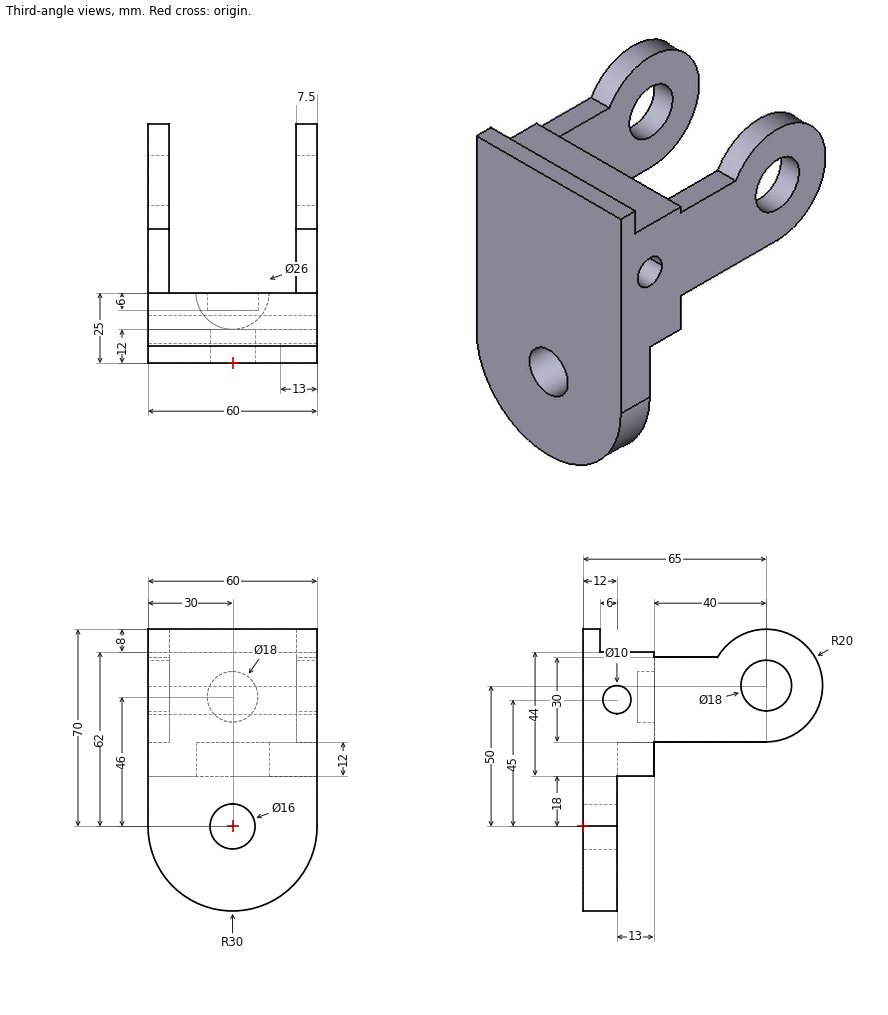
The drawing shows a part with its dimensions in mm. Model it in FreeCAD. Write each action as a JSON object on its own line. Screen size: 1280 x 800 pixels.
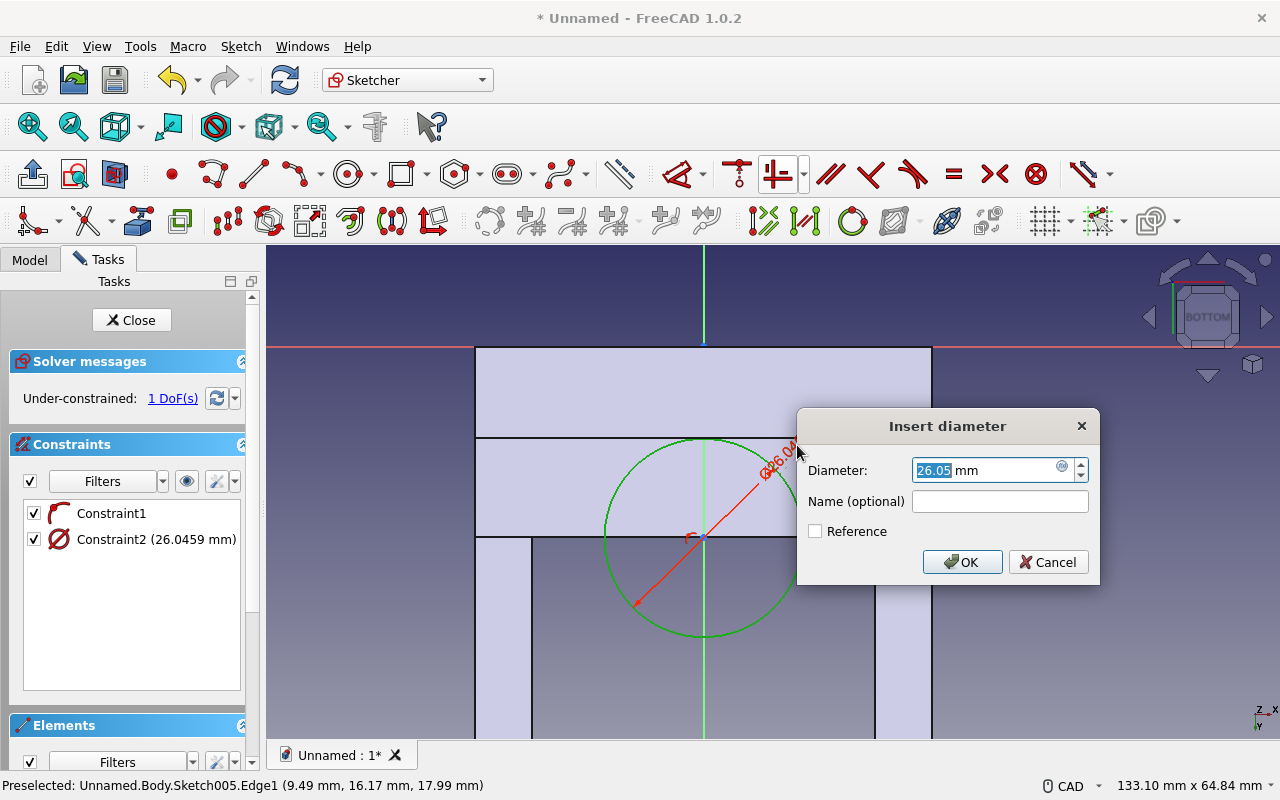
{"action": "type", "text": "26"}
{"action": "key", "text": "Return"}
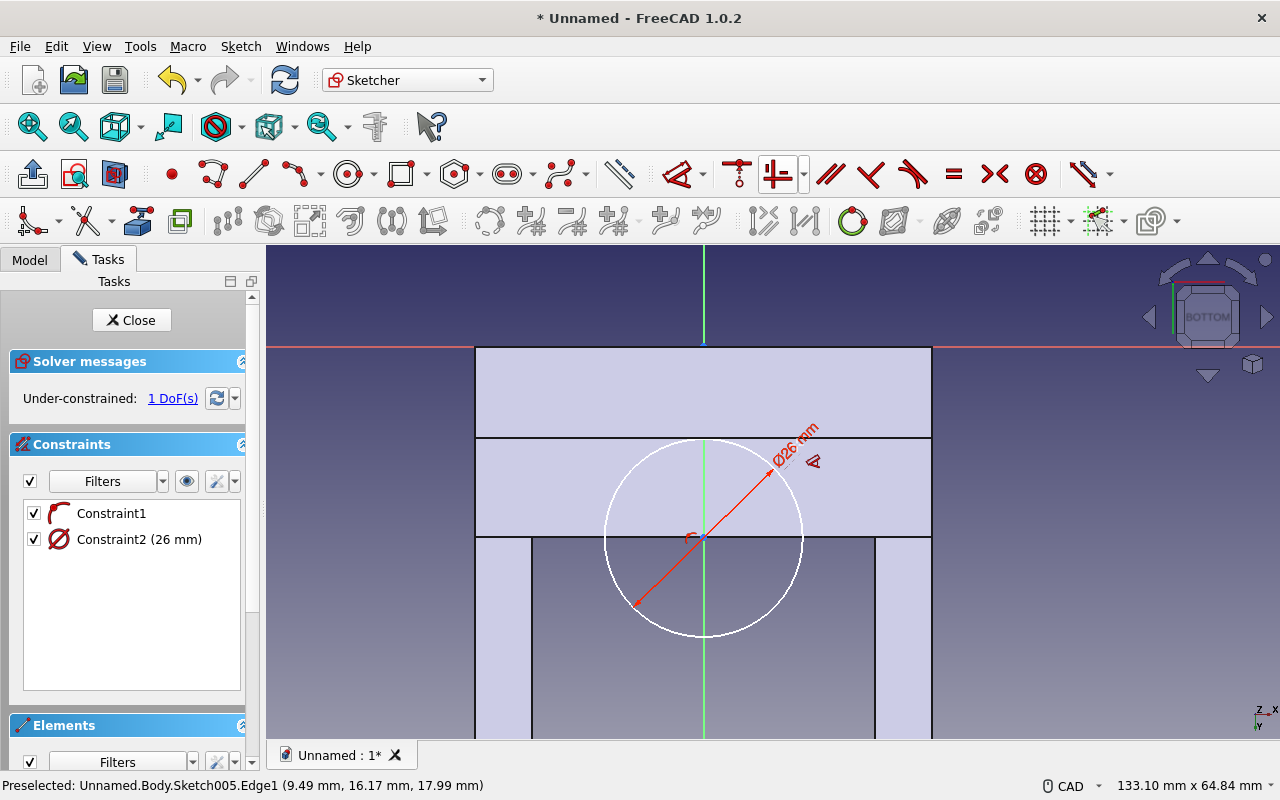
{"action": "left_click", "coordinate": [704, 538]}
{"action": "left_click", "coordinate": [738, 398]}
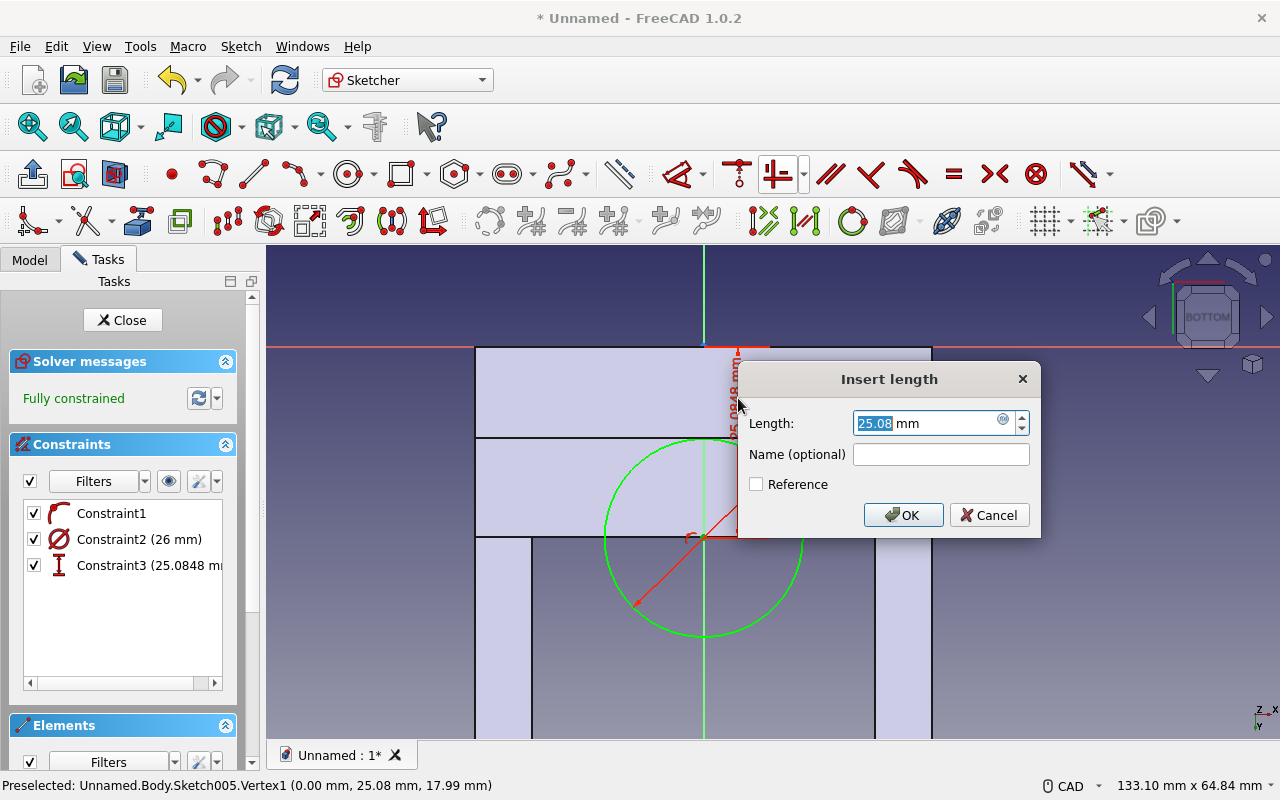
{"action": "type", "text": "25"}
{"action": "key", "text": "Return"}
{"action": "key", "text": "Escape"}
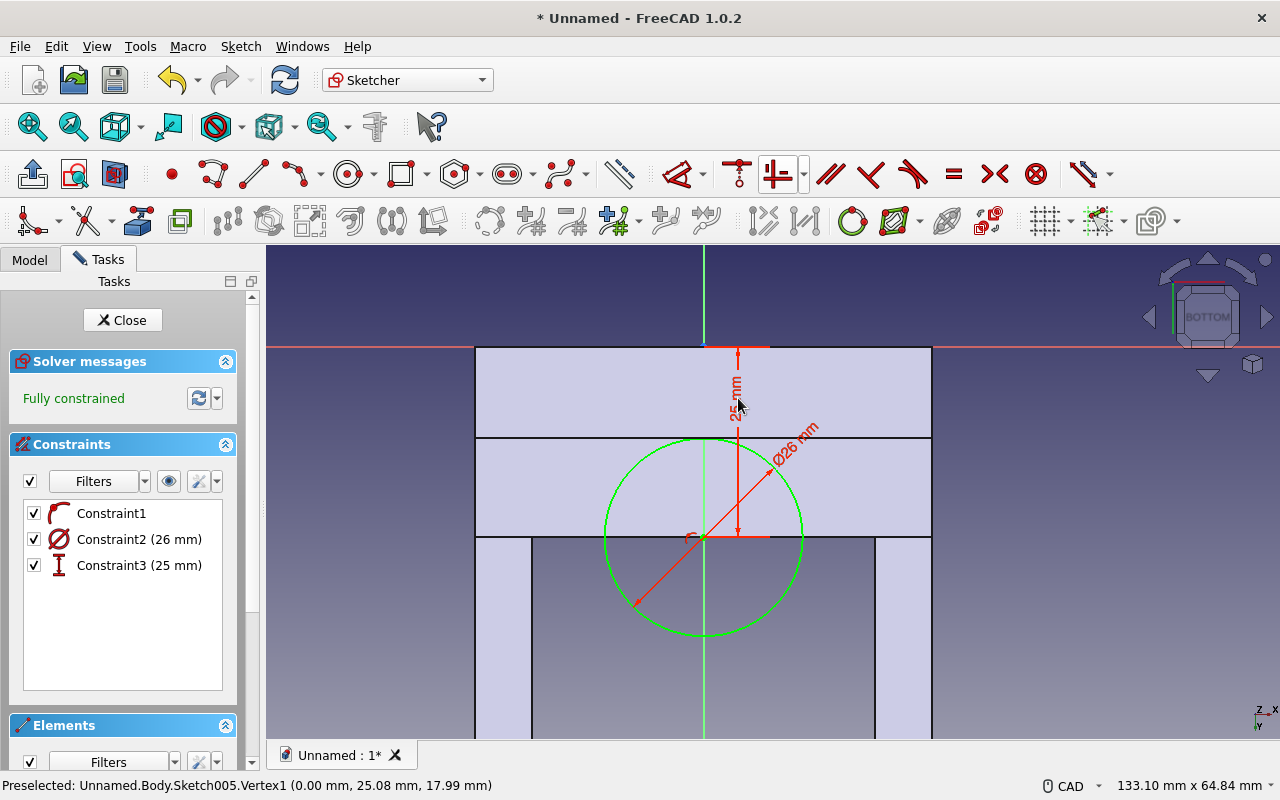
{"action": "left_click", "coordinate": [123, 320]}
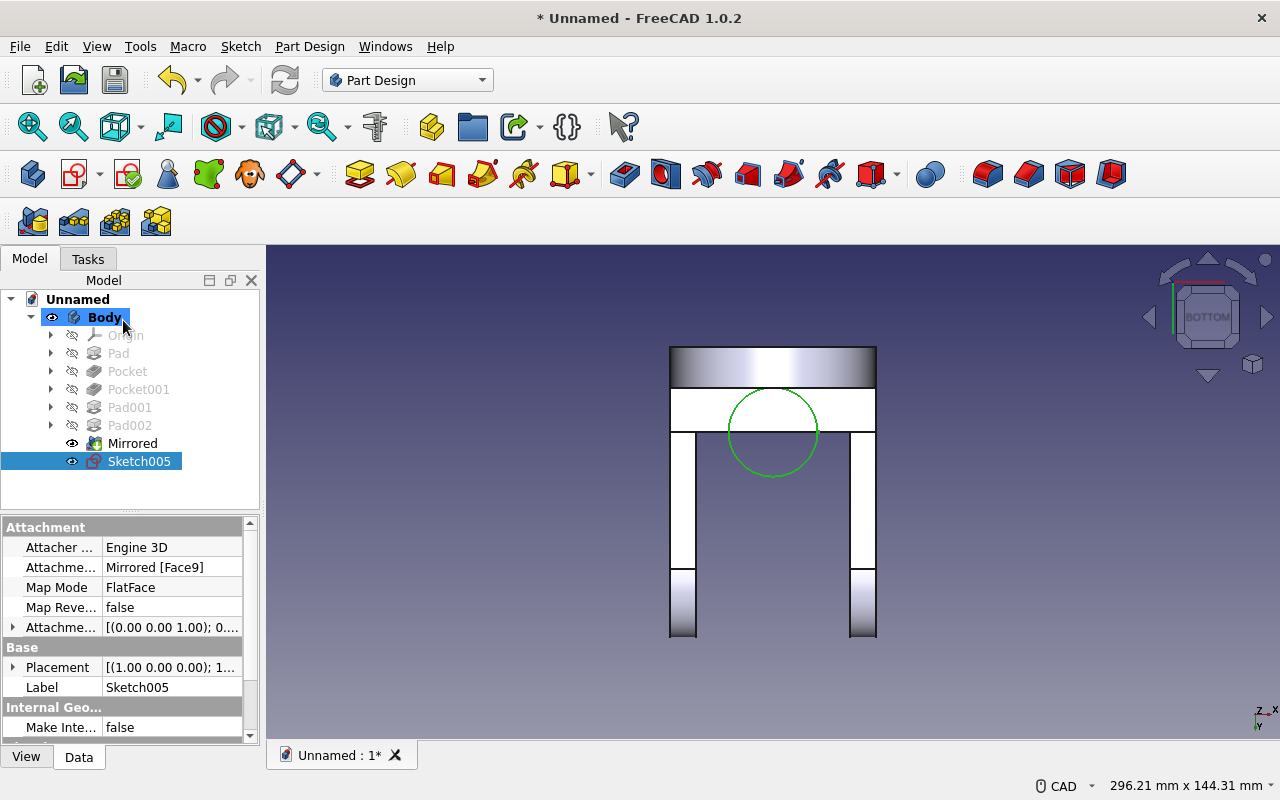
{"action": "left_click", "coordinate": [625, 174]}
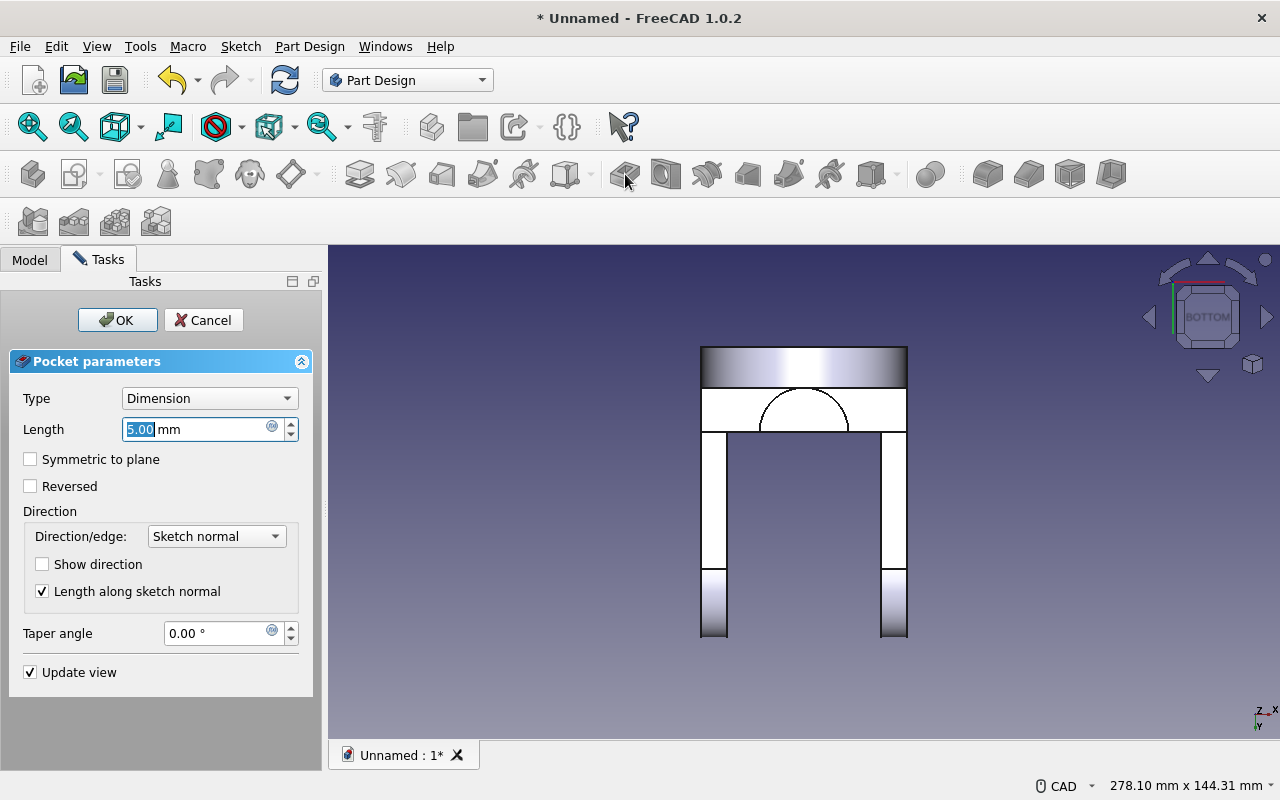
{"action": "type", "text": "12"}
{"action": "key", "text": "Tab"}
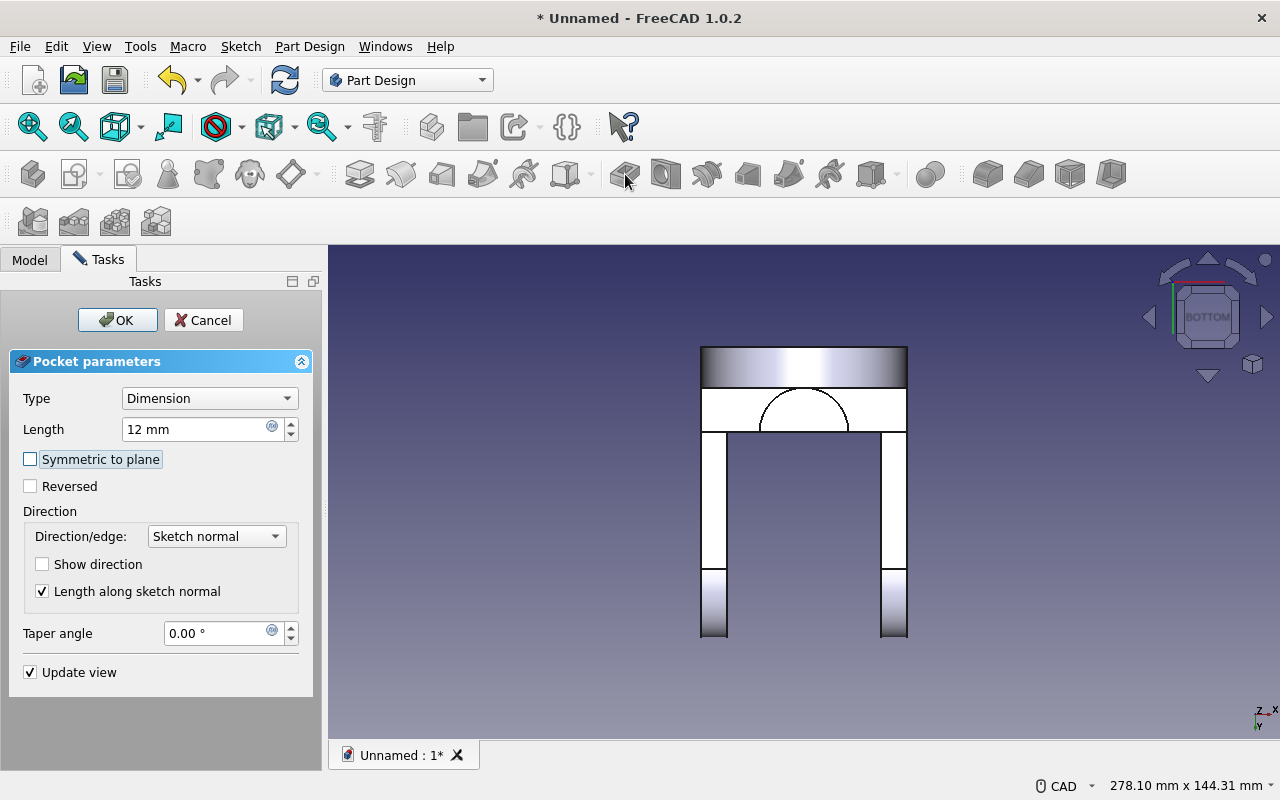
{"action": "left_click", "coordinate": [118, 320]}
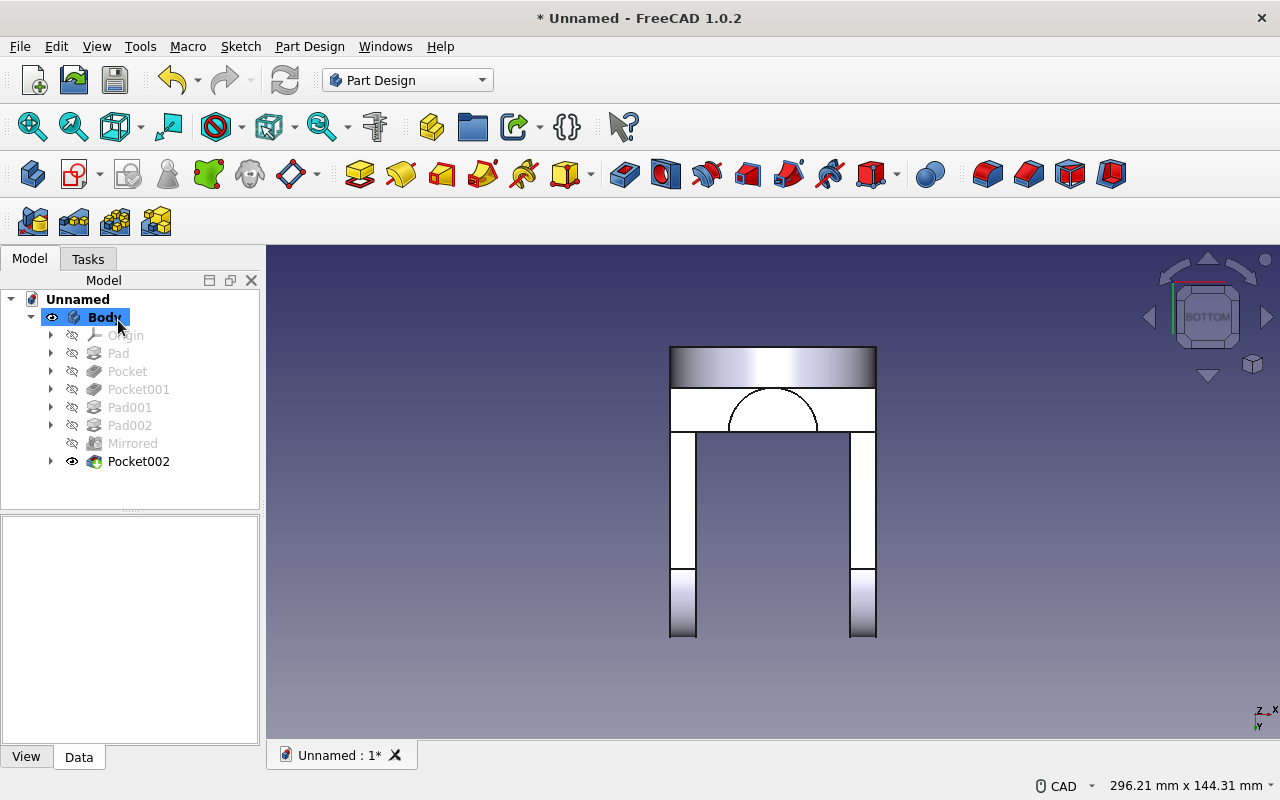
{"action": "key", "text": "4"}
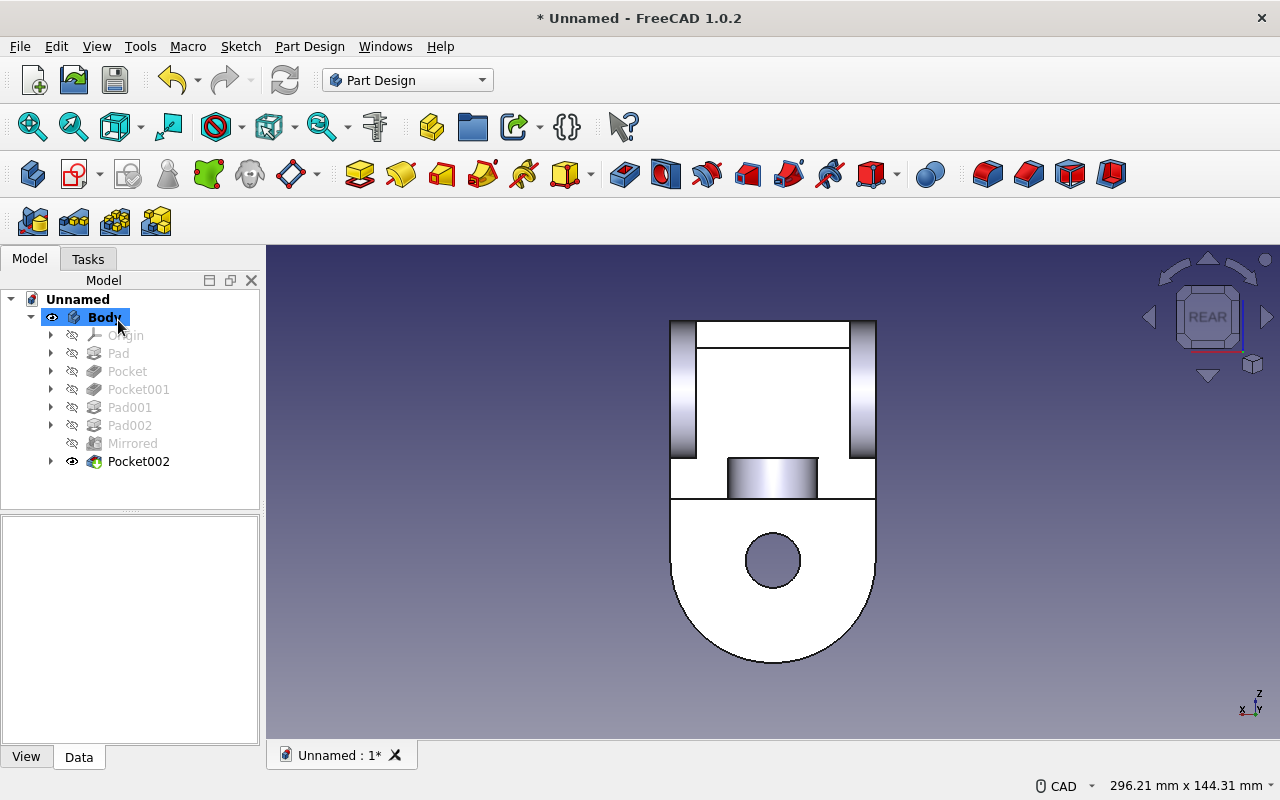
{"action": "left_click", "coordinate": [773, 401]}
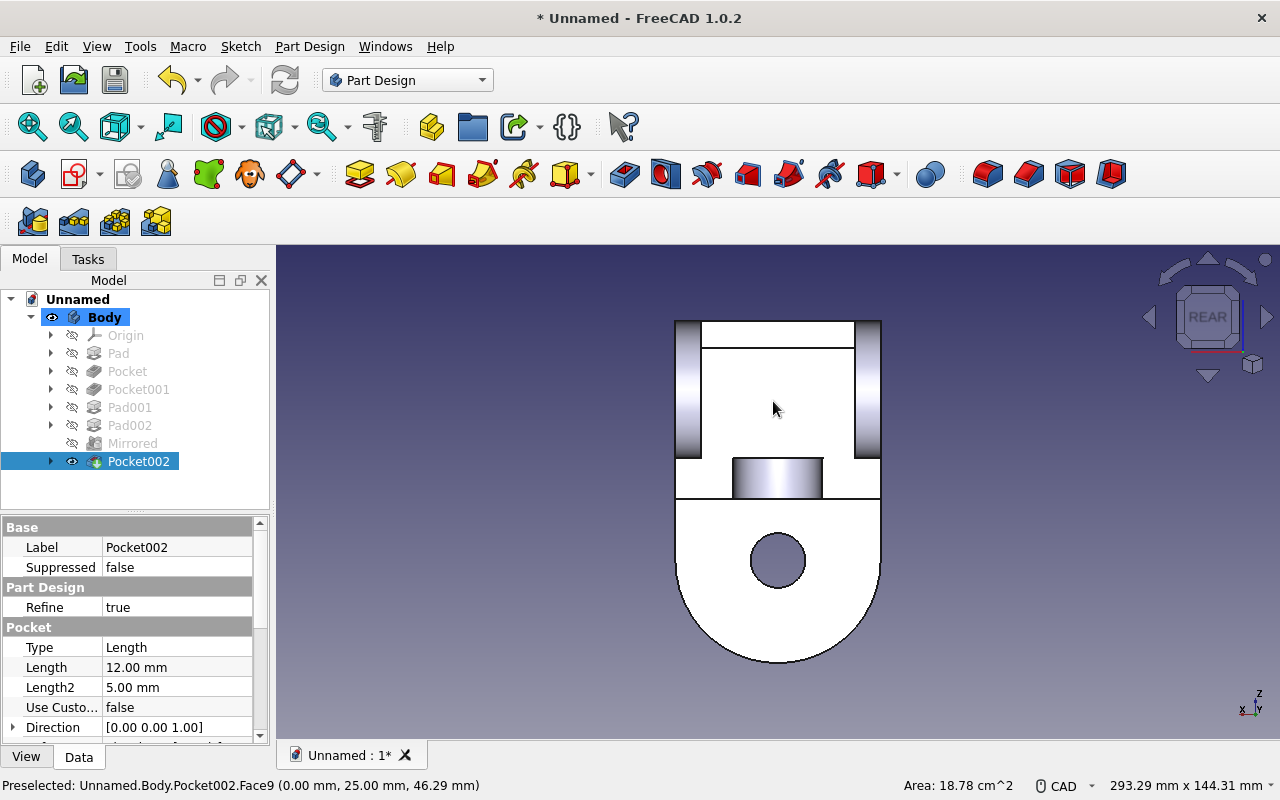
{"action": "left_click", "coordinate": [74, 174]}